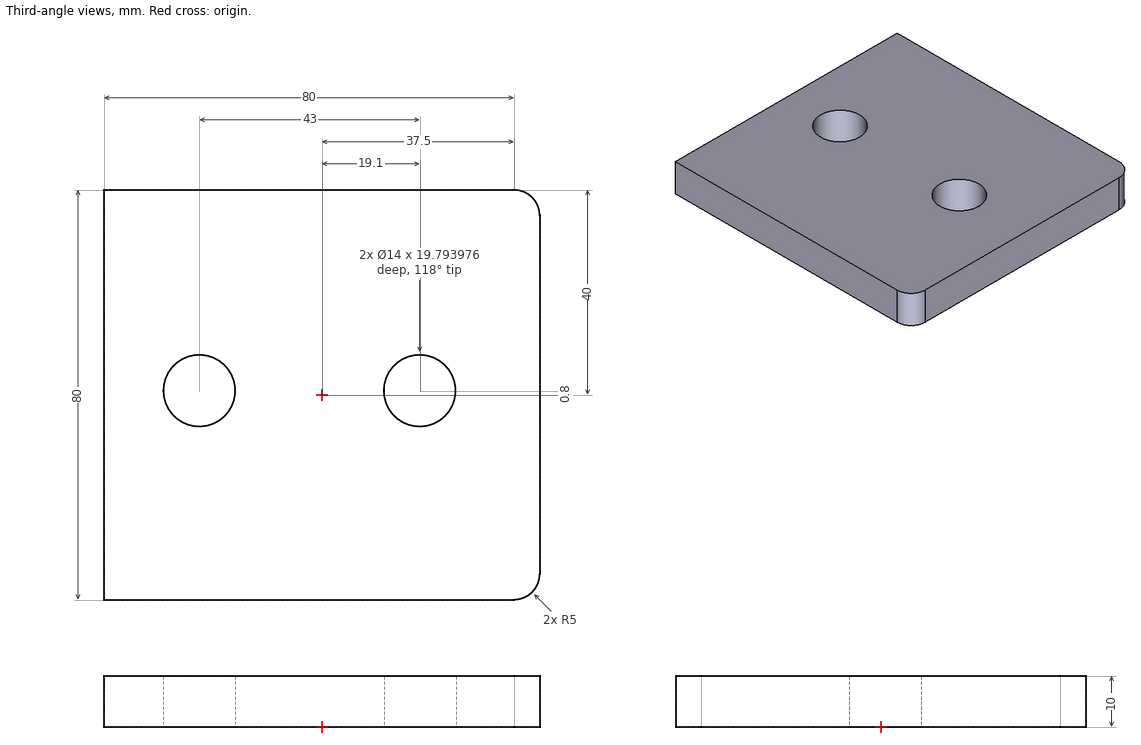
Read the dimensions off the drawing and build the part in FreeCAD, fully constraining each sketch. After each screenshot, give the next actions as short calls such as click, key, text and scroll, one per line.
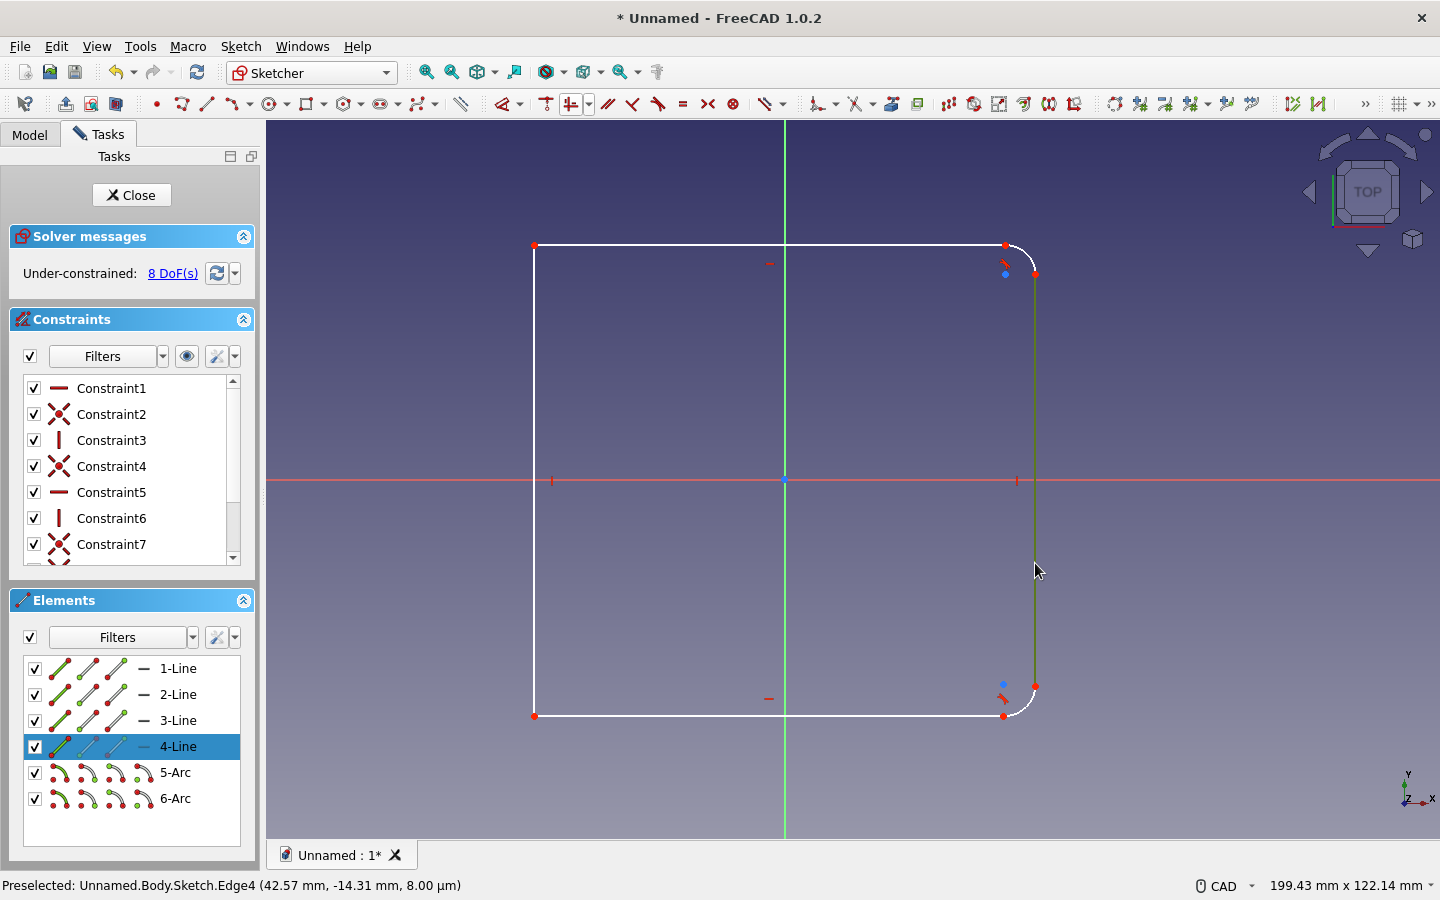
click(1018, 713)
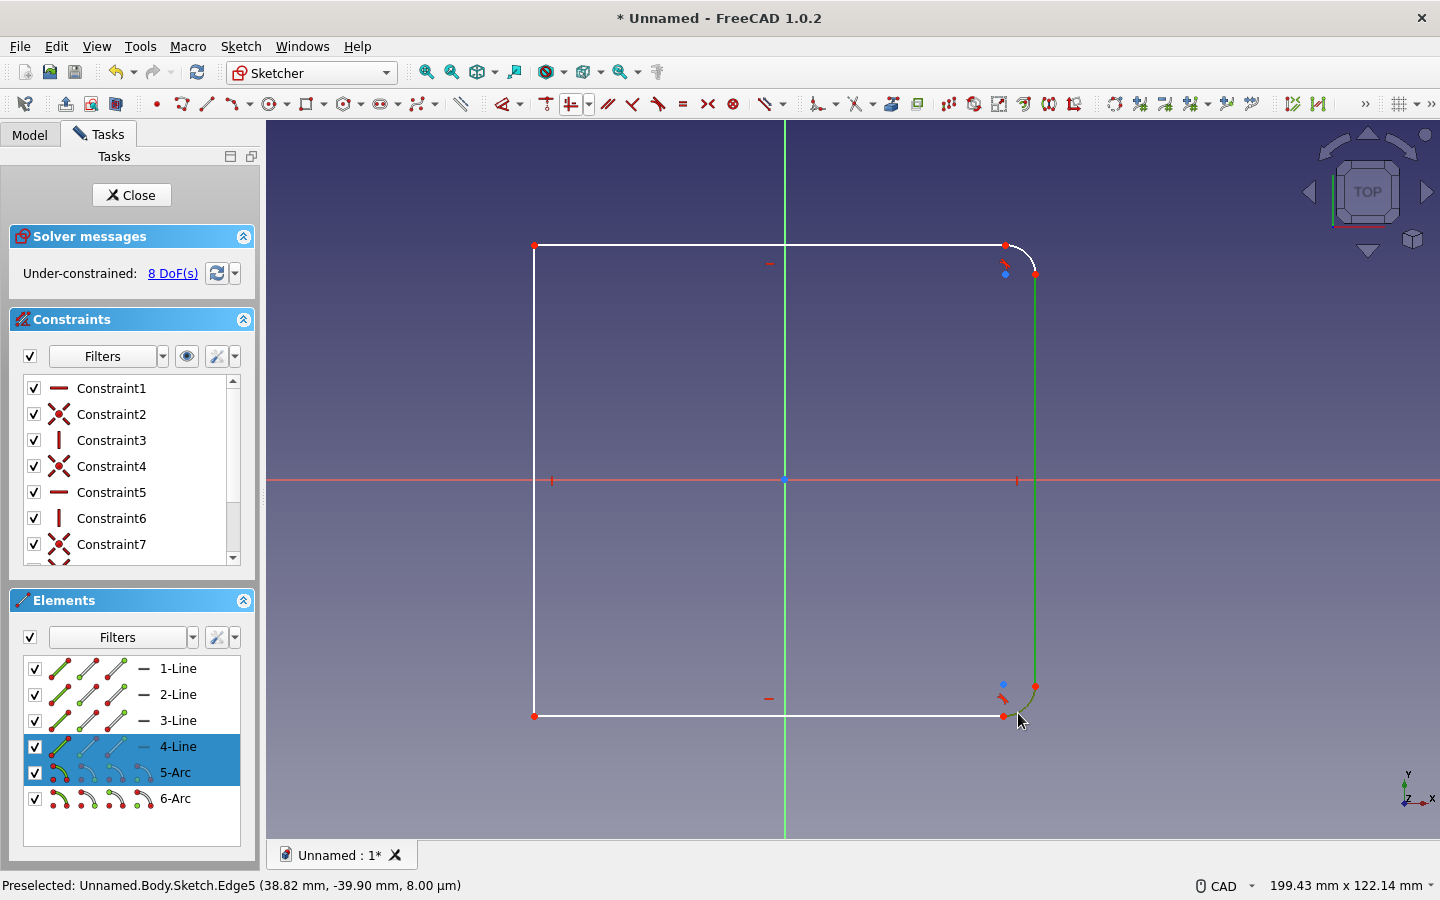
click(658, 104)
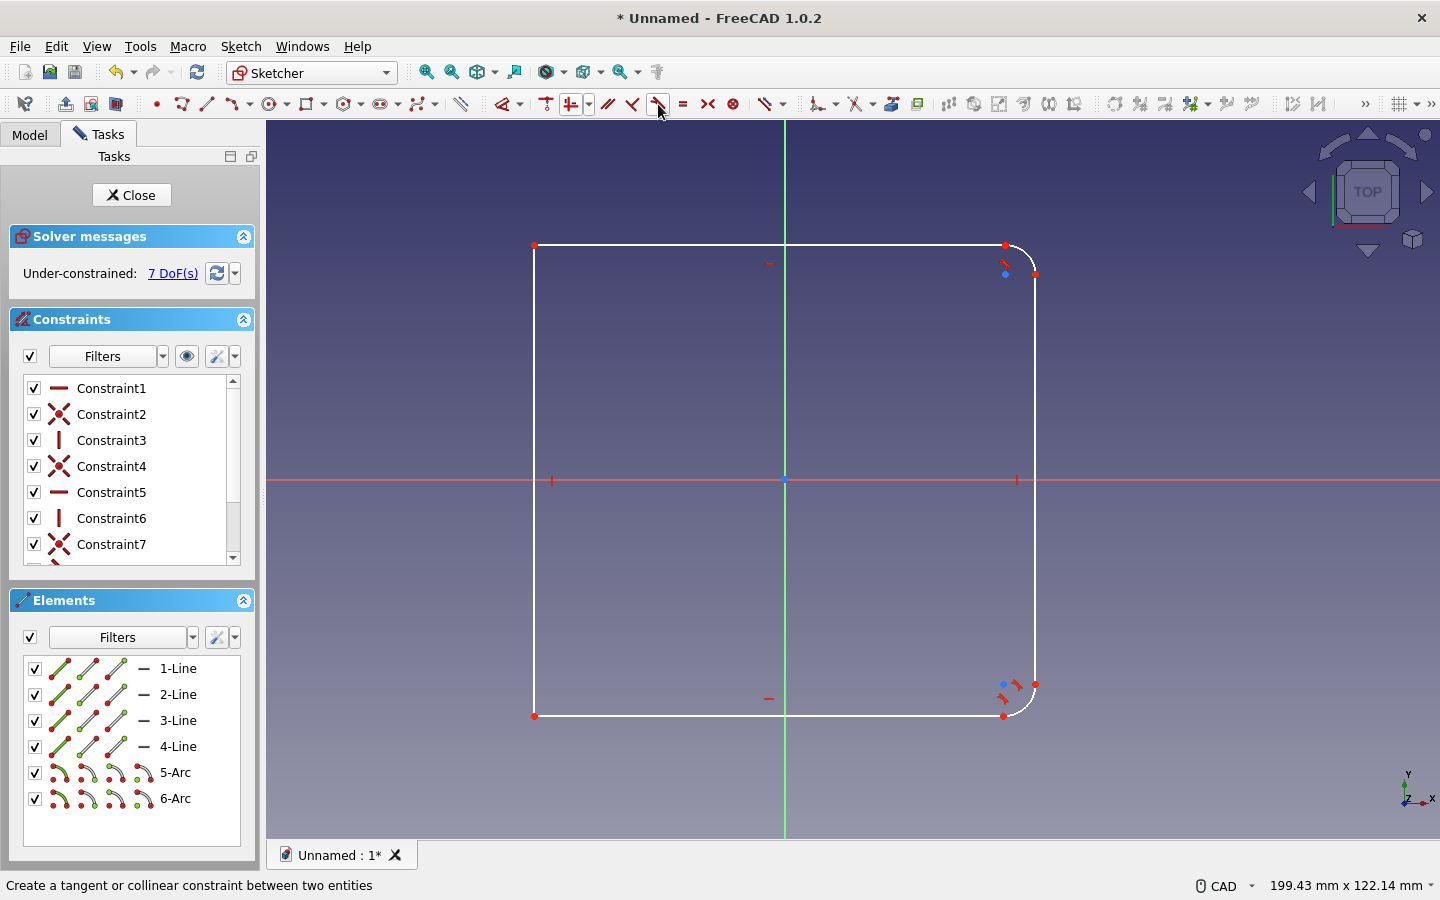
click(1035, 562)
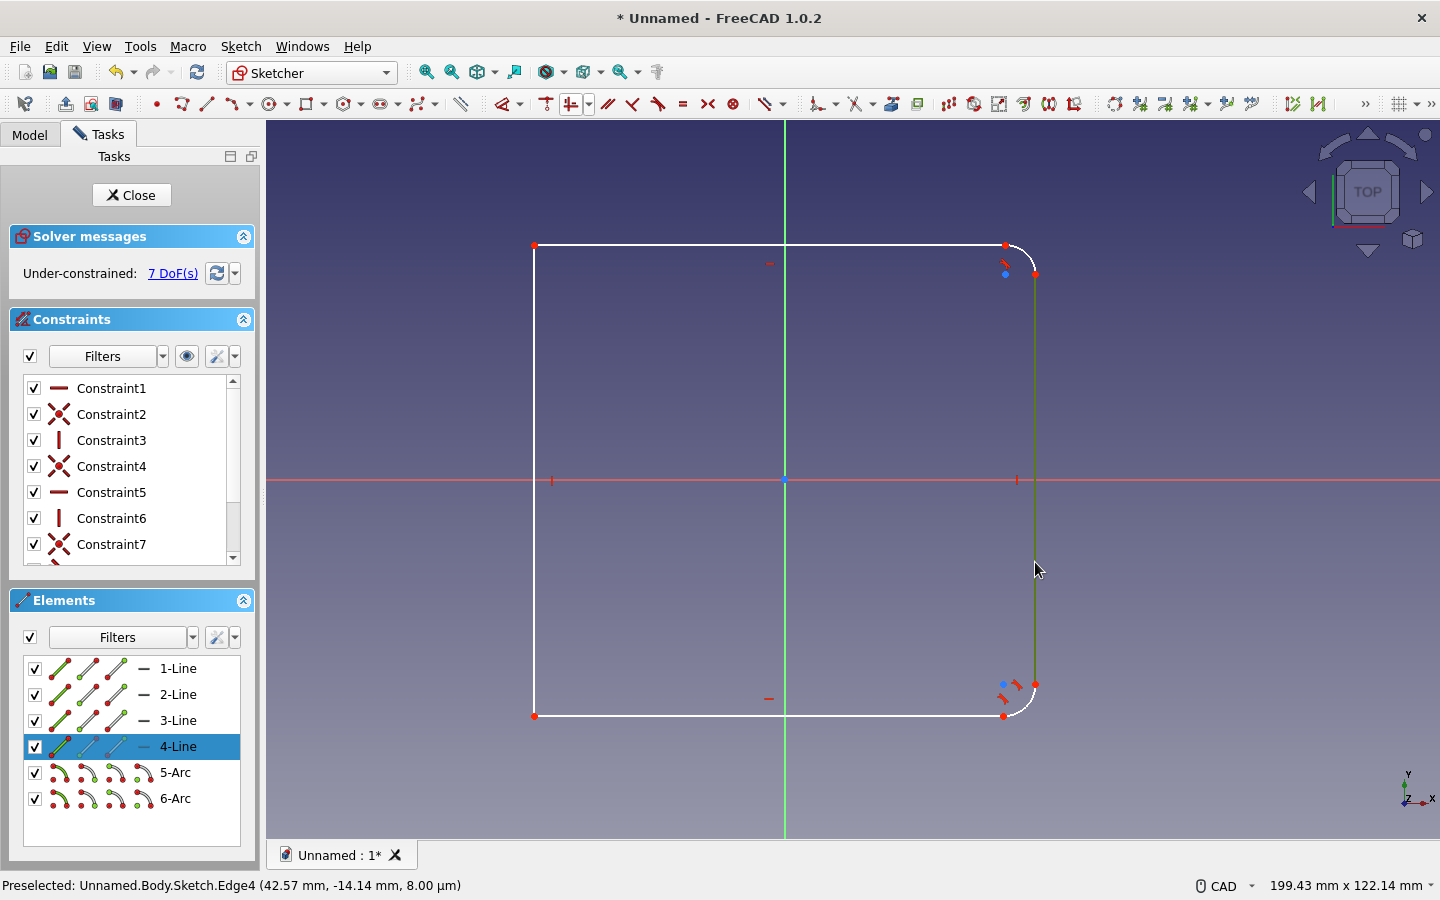
click(1032, 261)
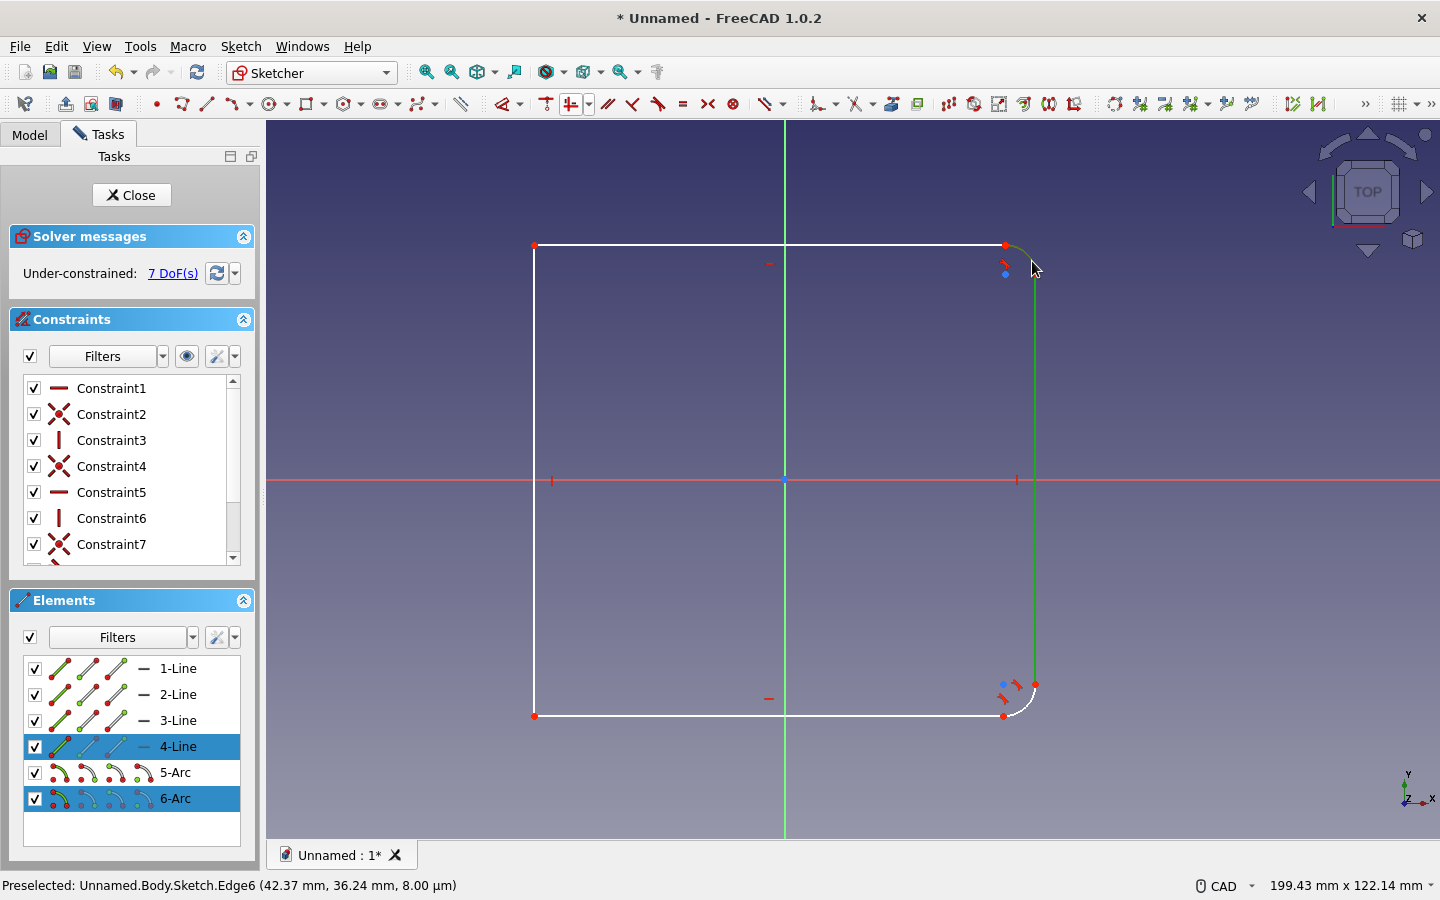
click(658, 104)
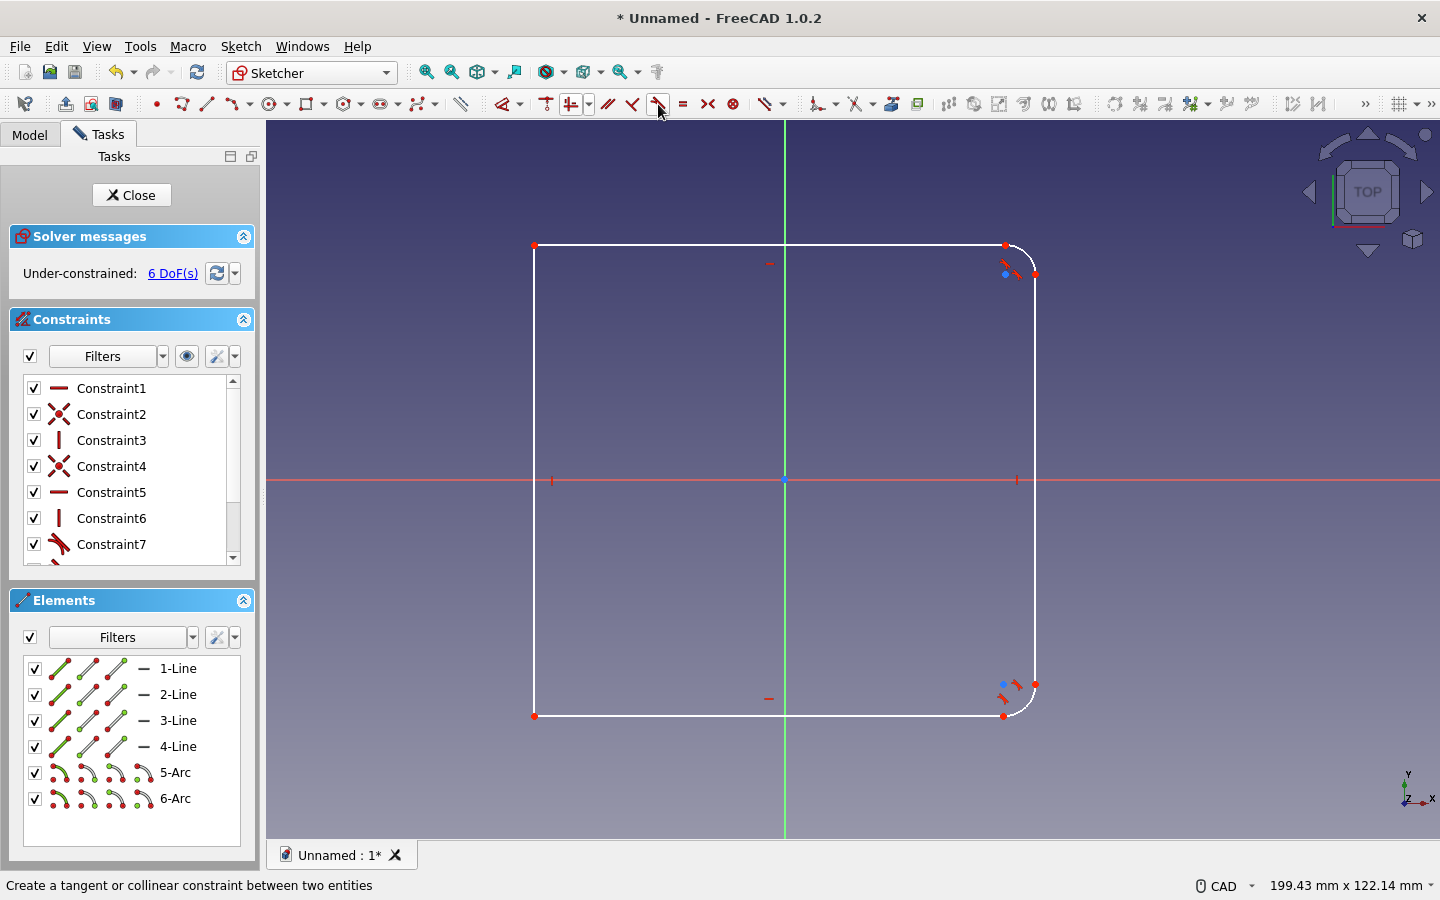
click(1018, 713)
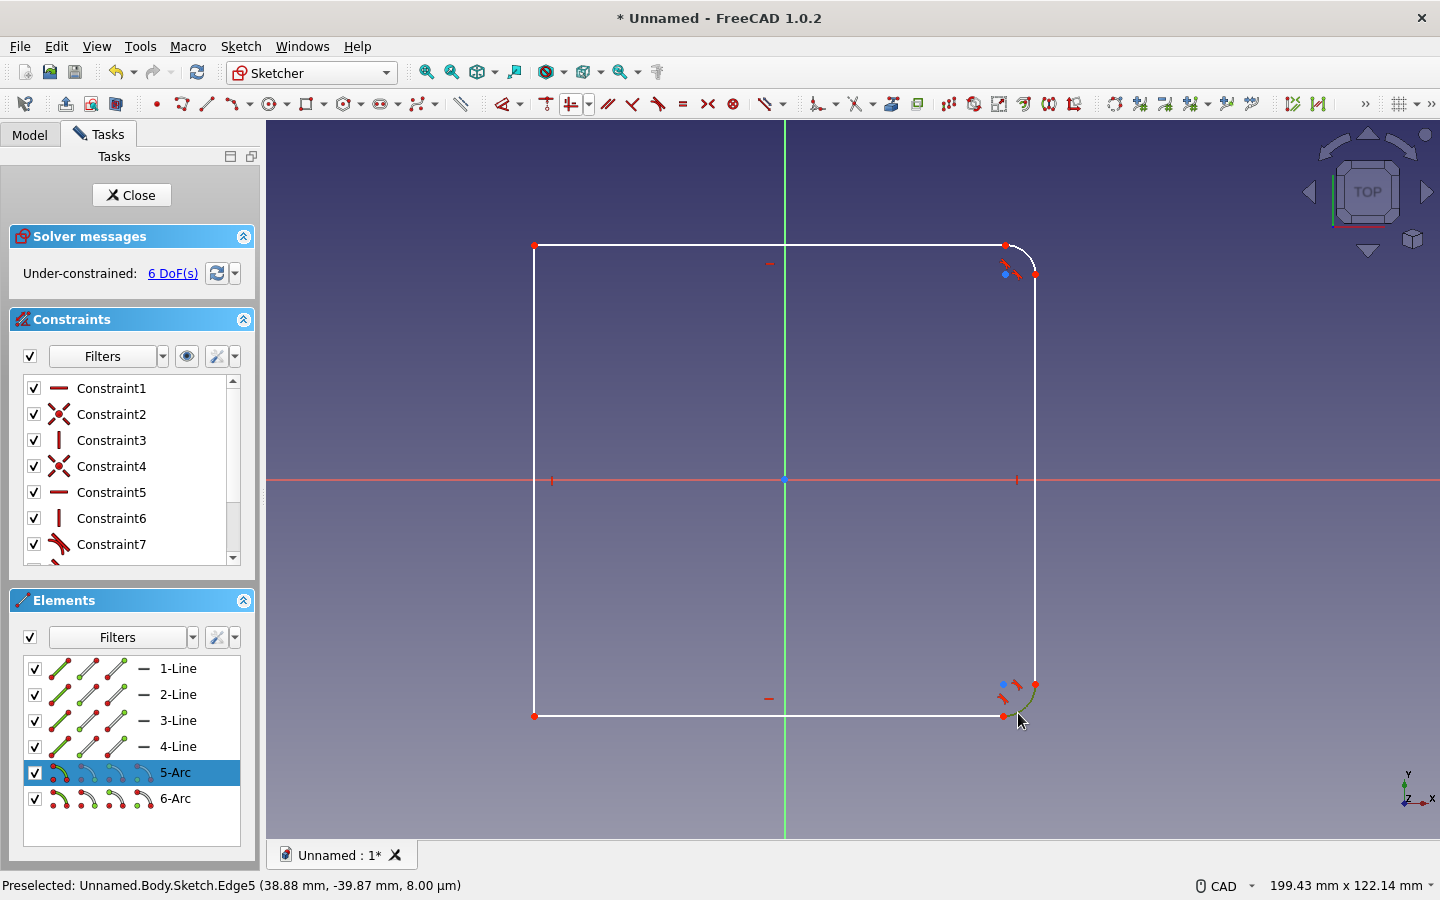
click(1032, 261)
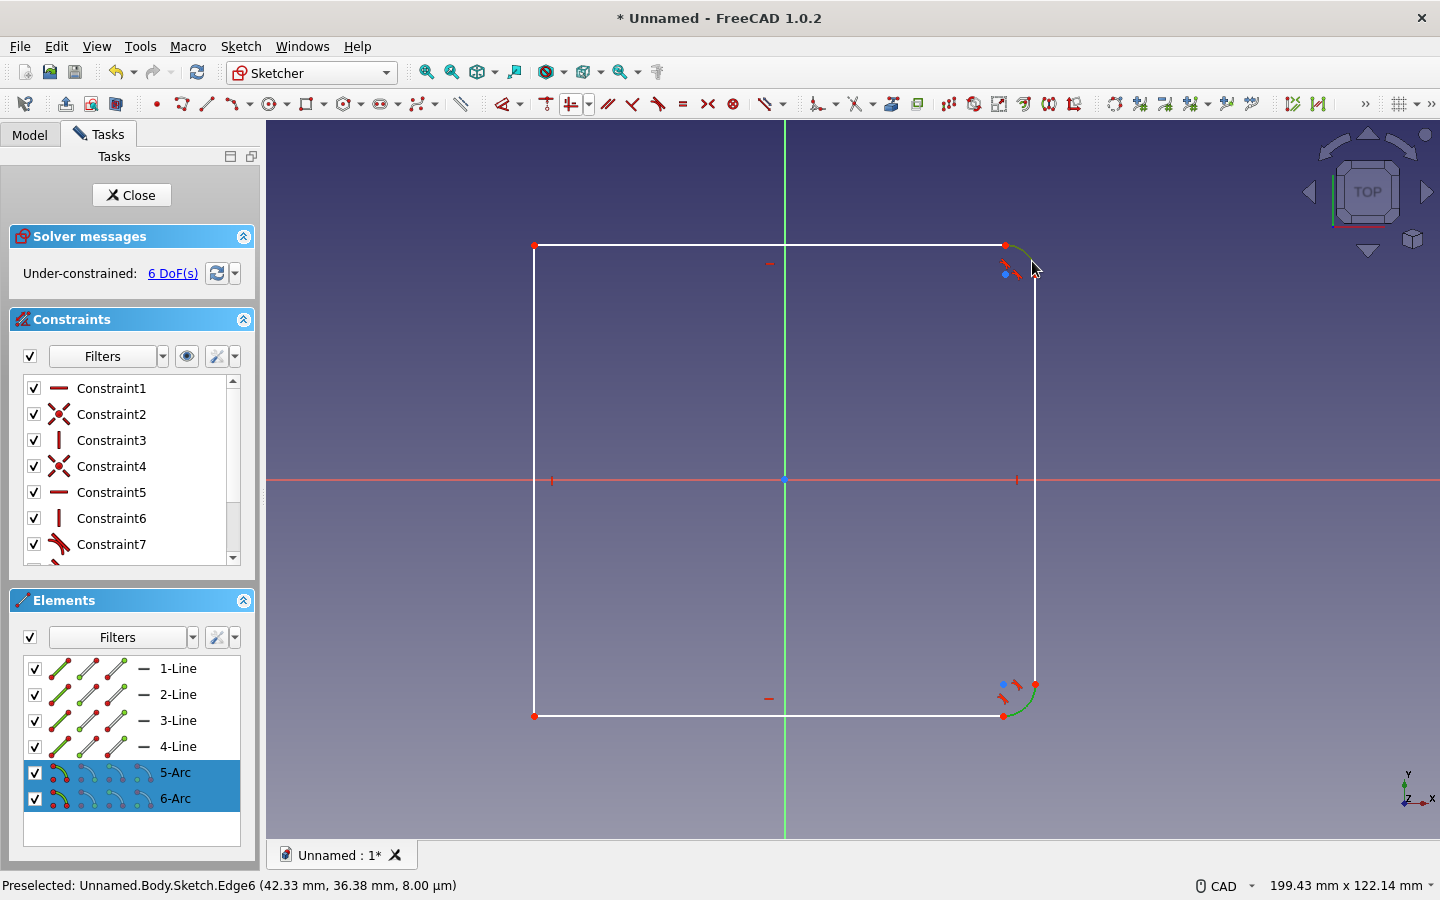
key(e)